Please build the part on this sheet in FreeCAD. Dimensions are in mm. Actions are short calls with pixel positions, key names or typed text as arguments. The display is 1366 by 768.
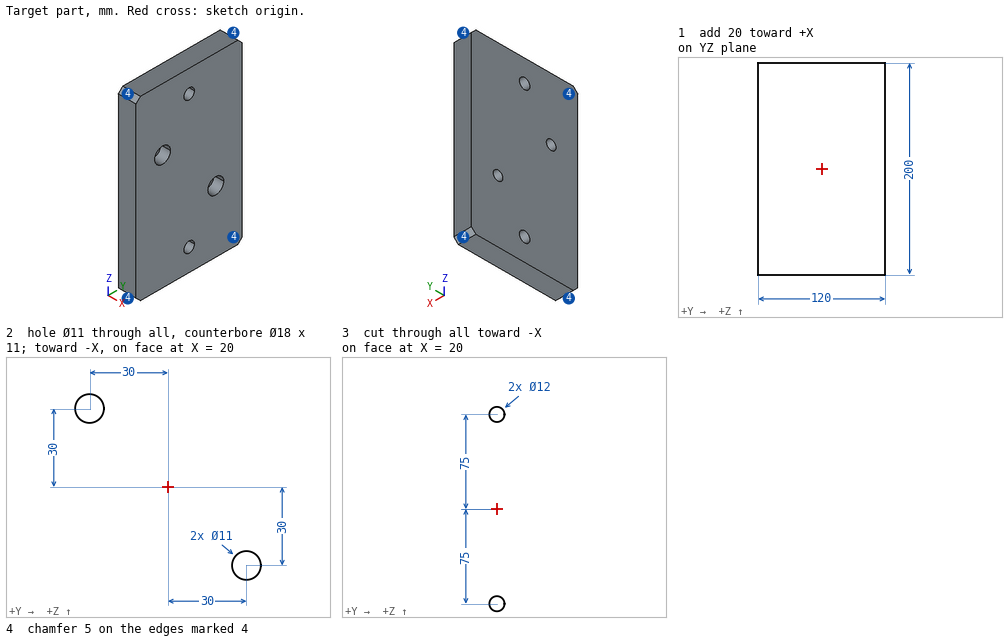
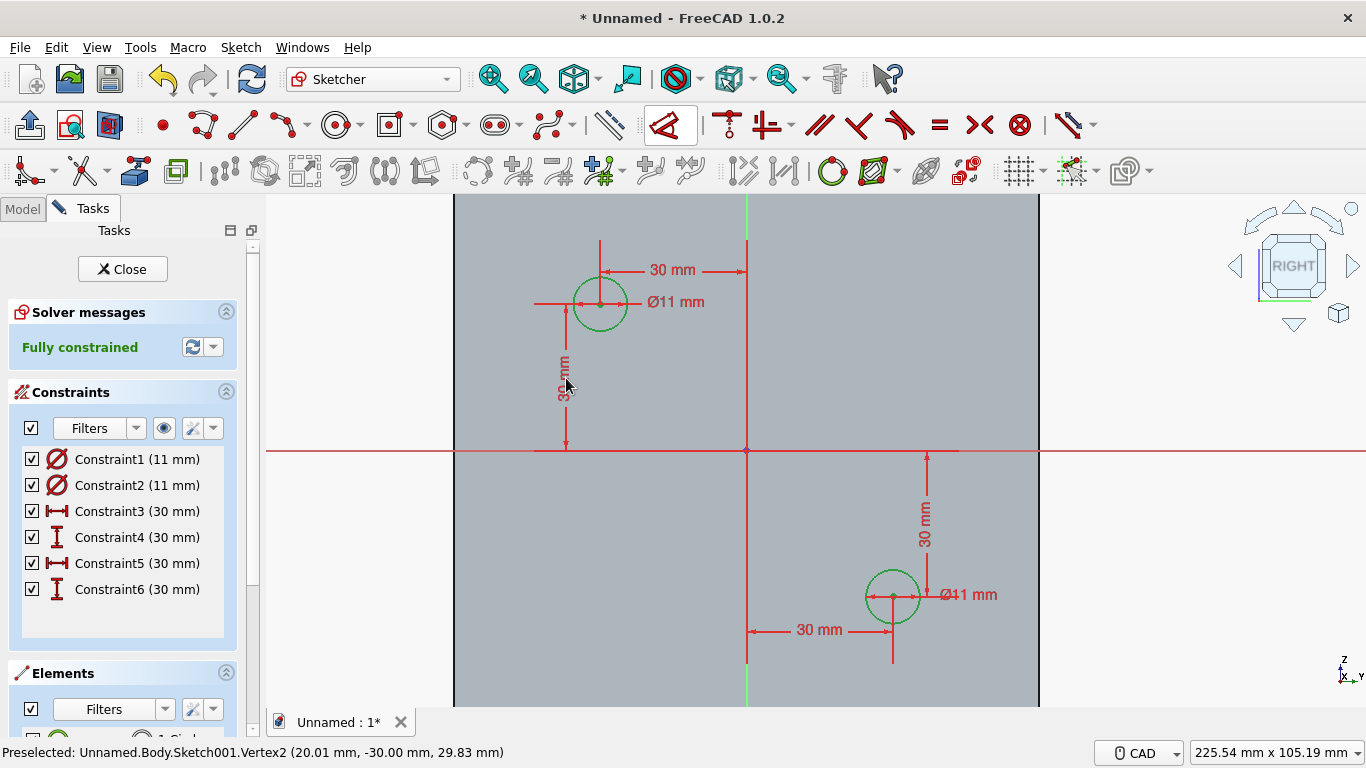
click(123, 269)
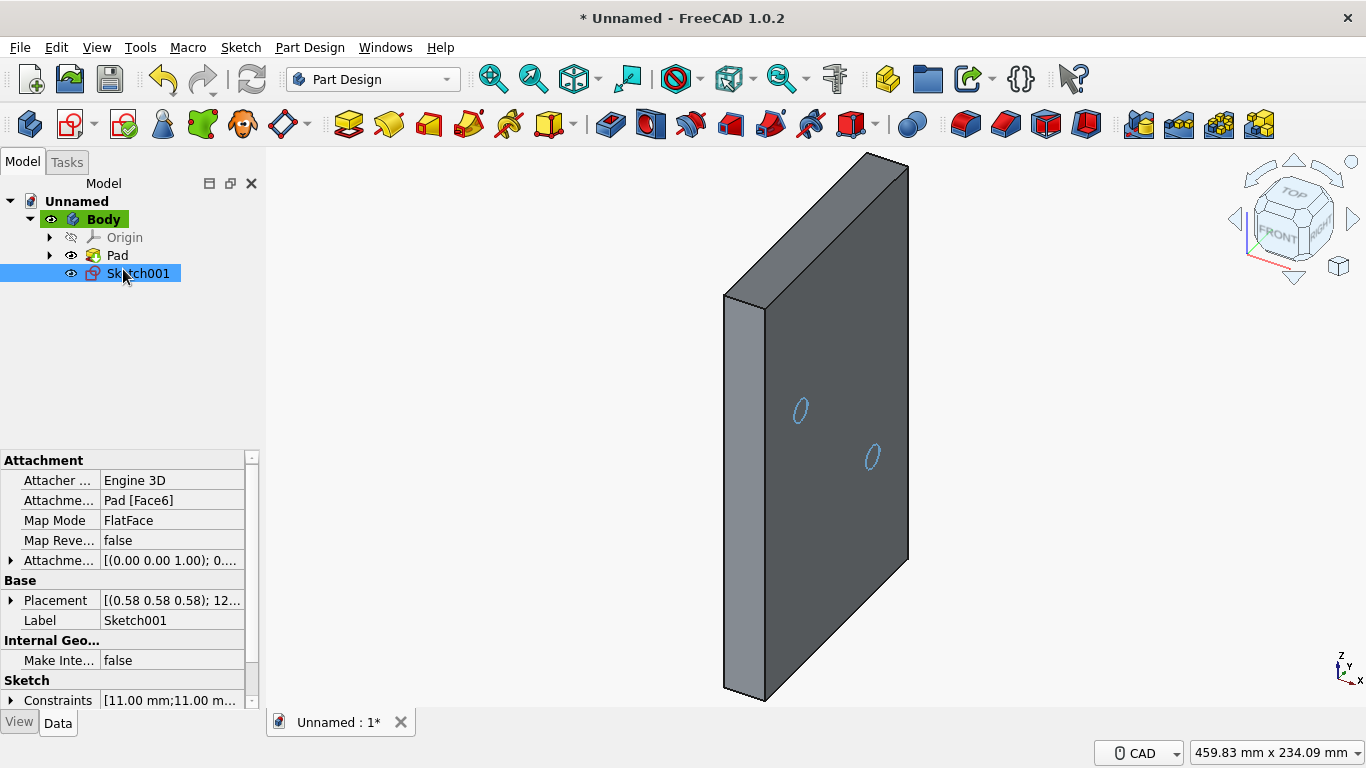
click(652, 124)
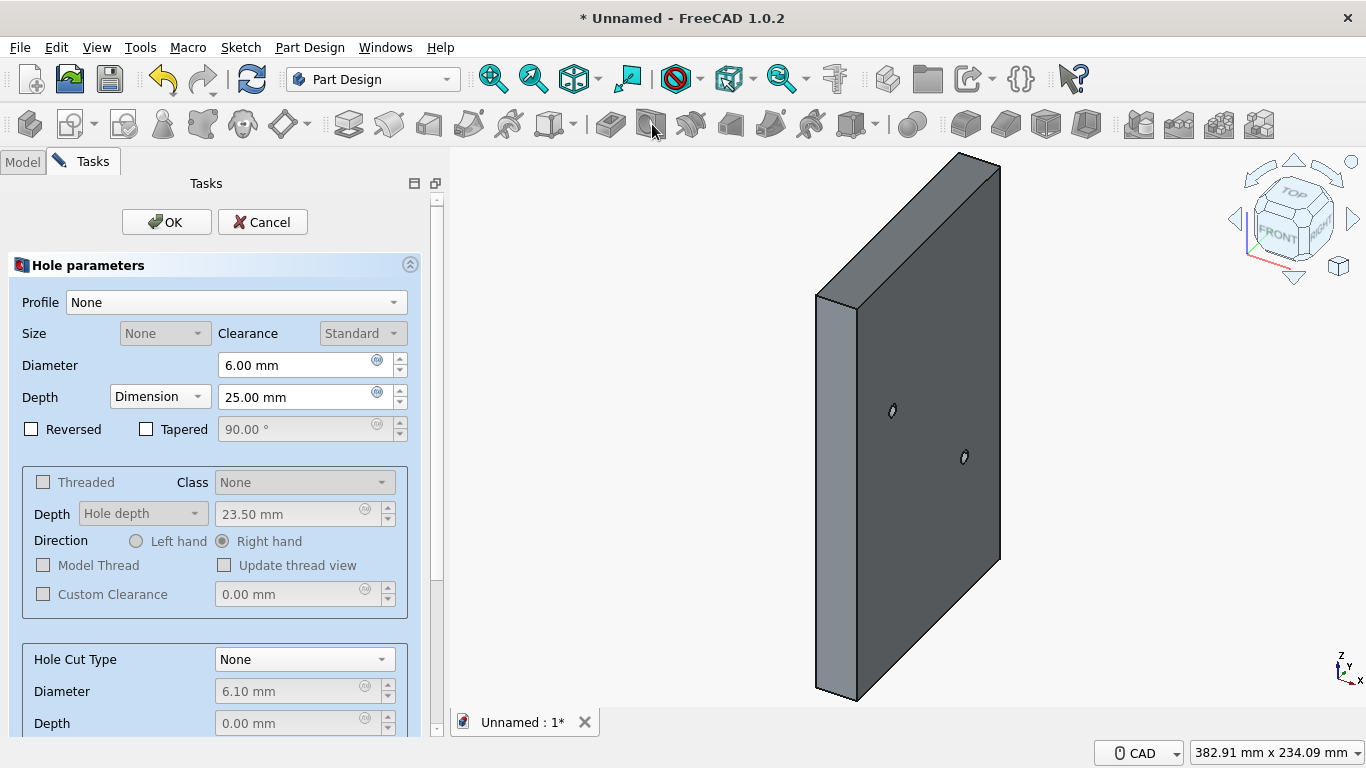
triple_click(305, 365)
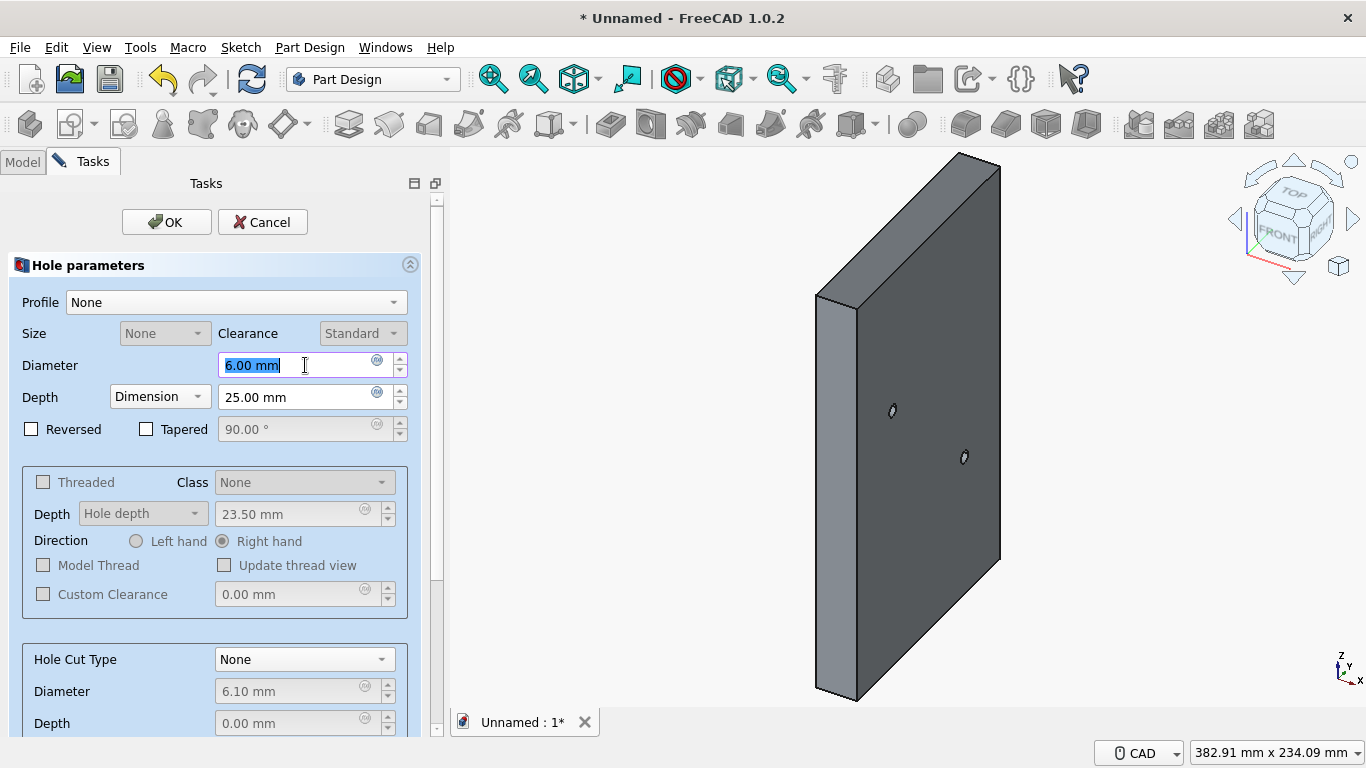
text(11)
key(Tab)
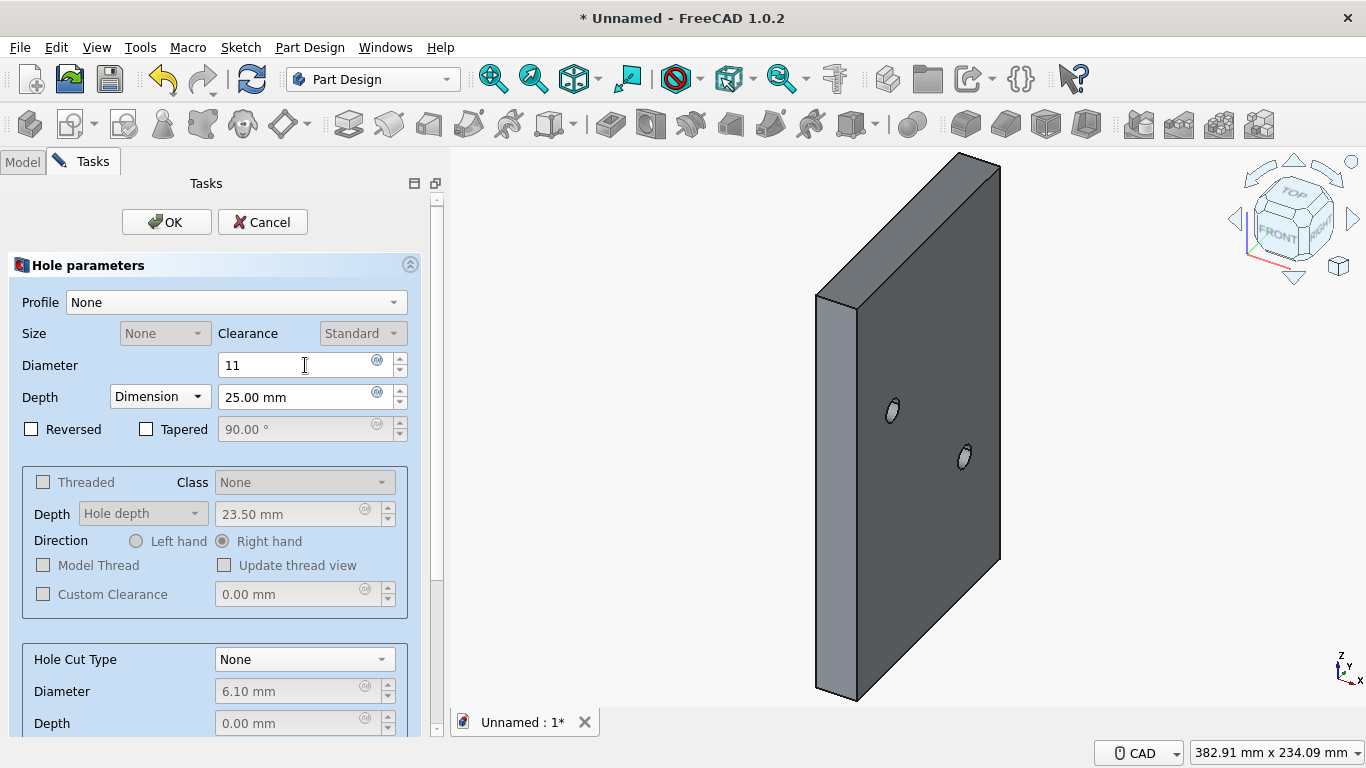
click(161, 396)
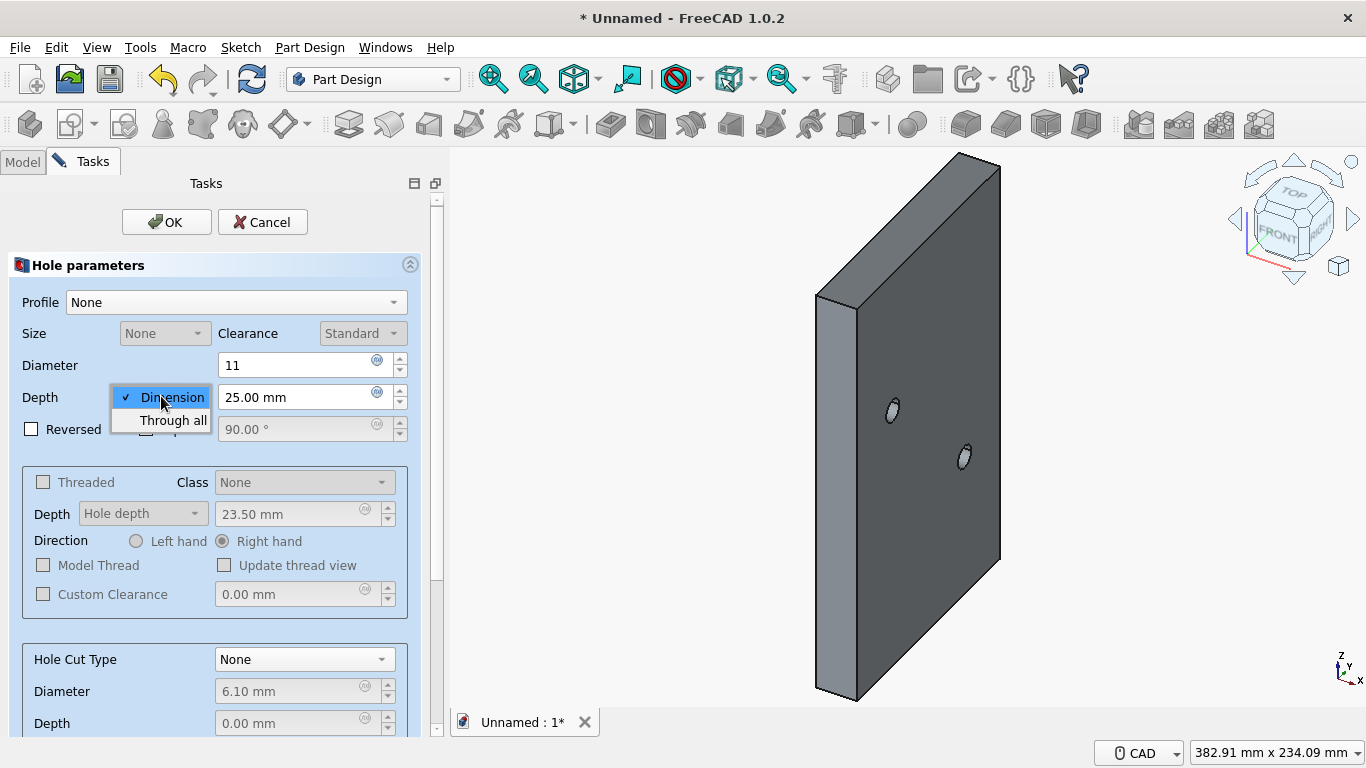
click(160, 420)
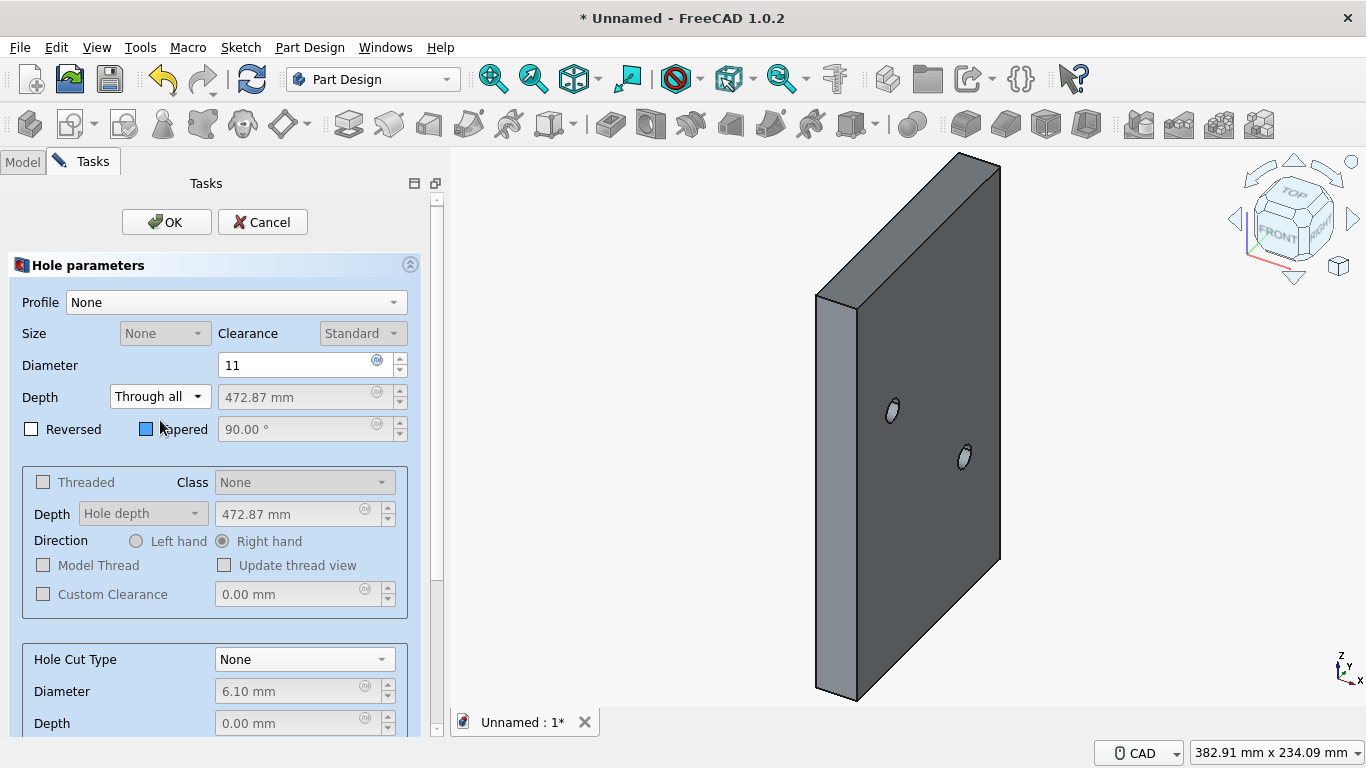
click(306, 660)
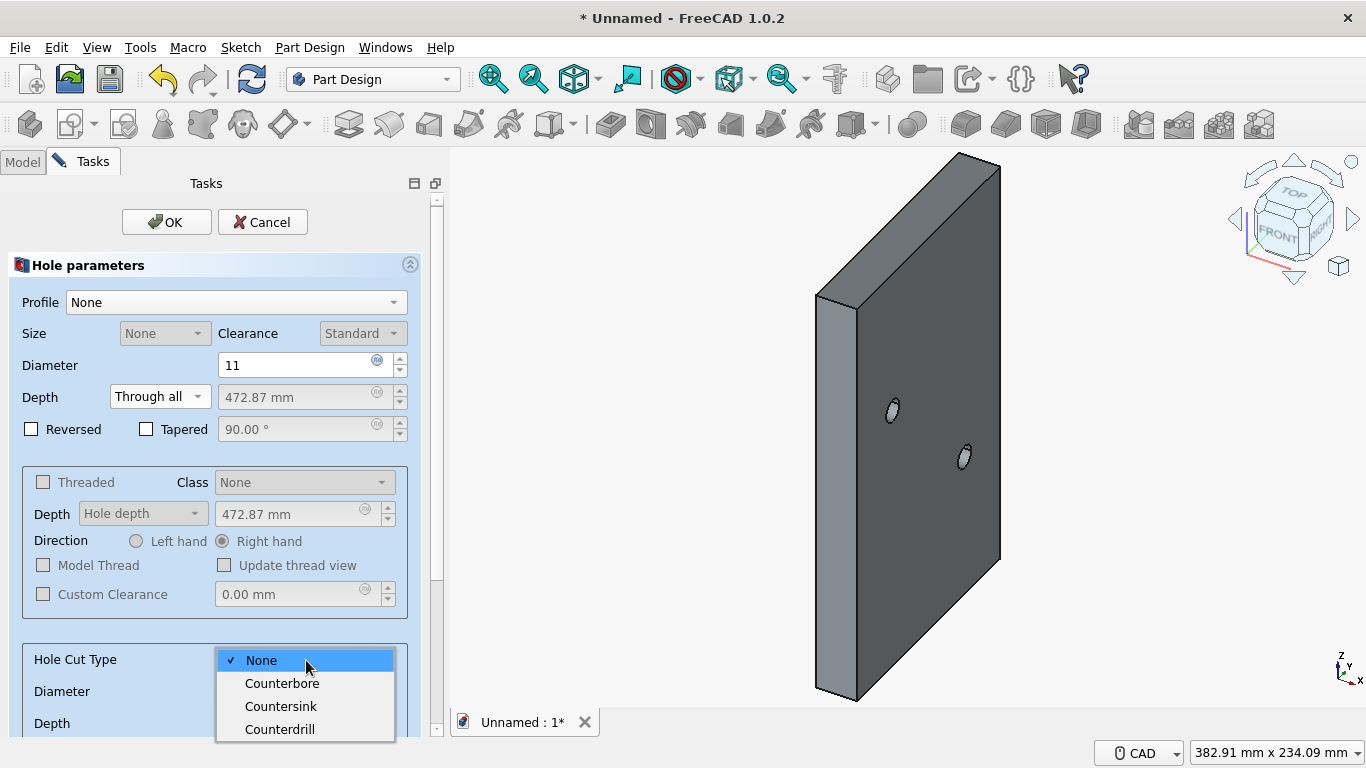
click(304, 684)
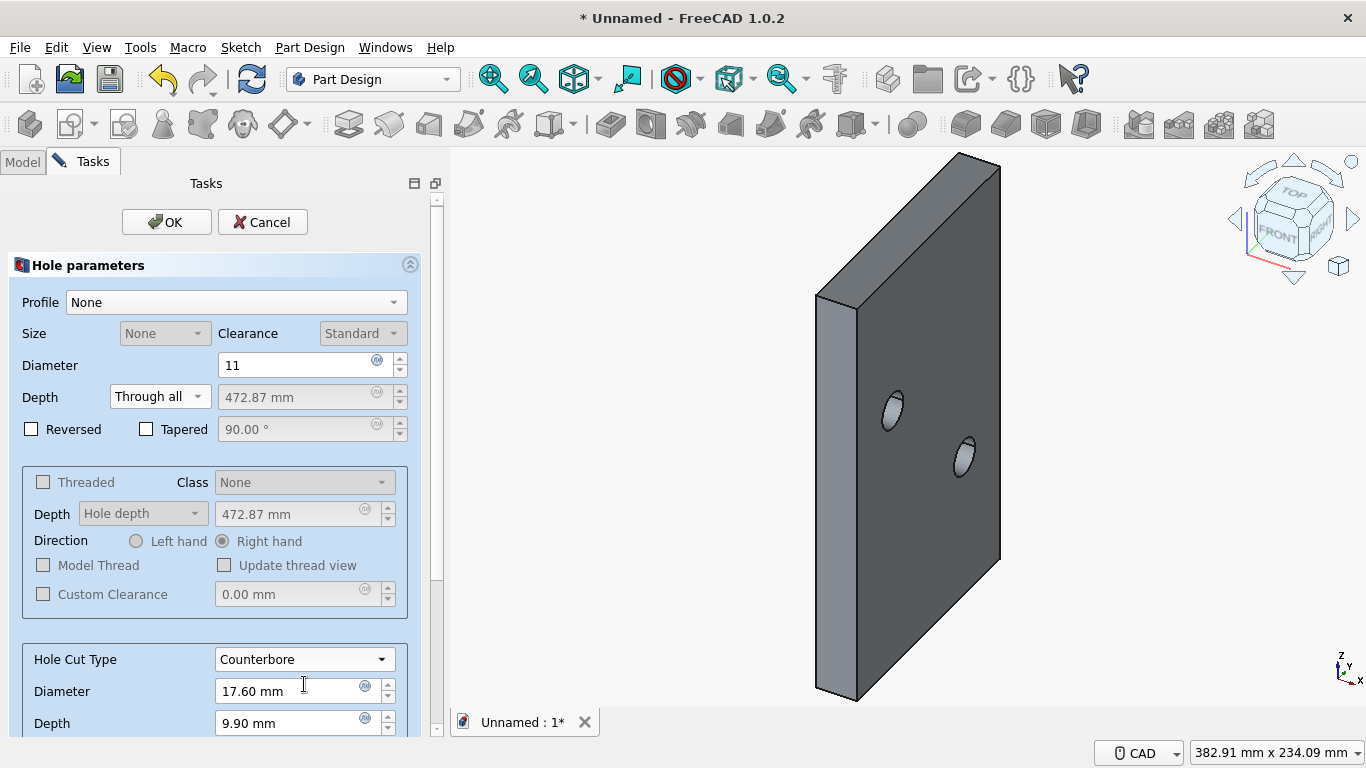
triple_click(298, 691)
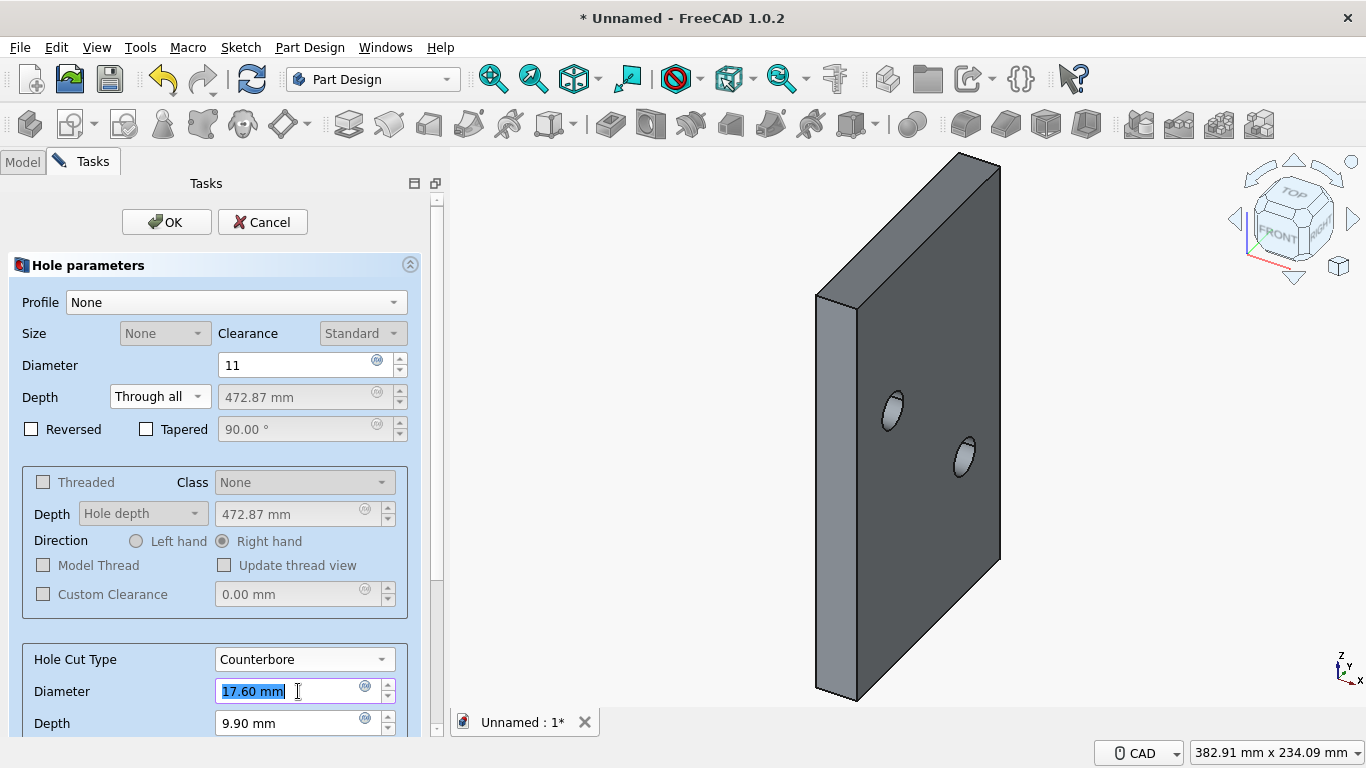
text(18)
key(Tab)